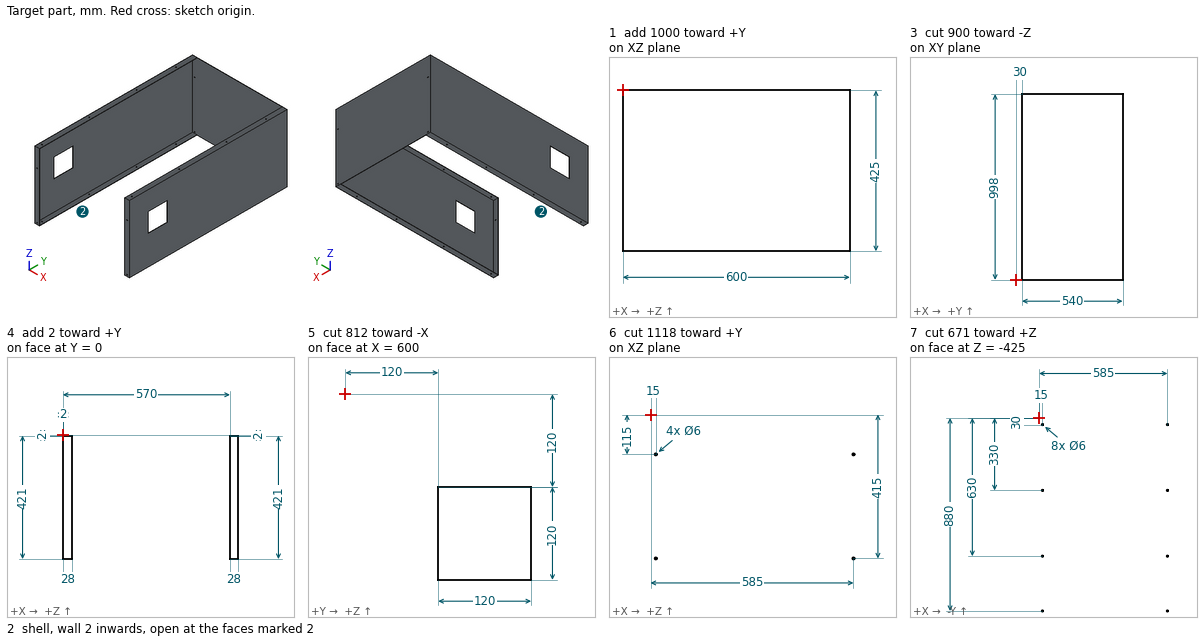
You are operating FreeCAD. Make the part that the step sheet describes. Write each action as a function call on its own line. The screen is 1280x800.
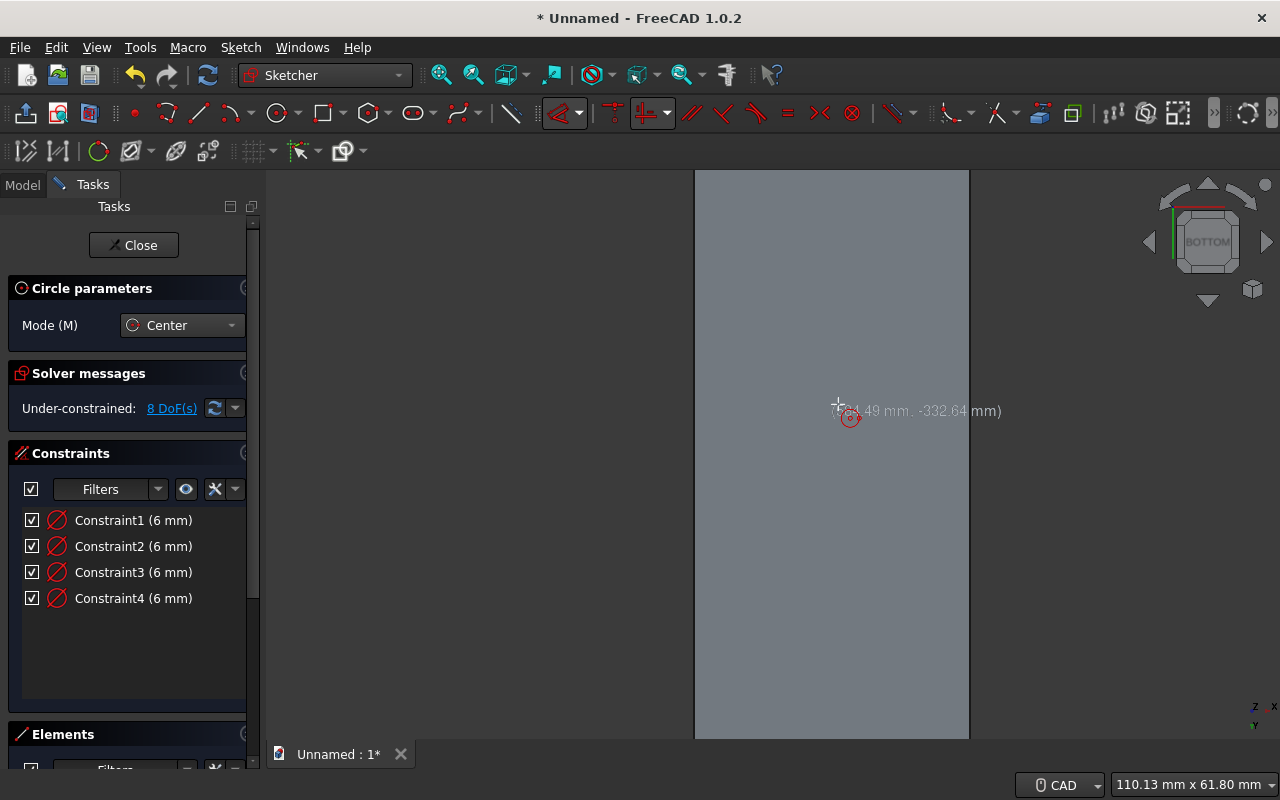
scroll(838, 404, down, 15)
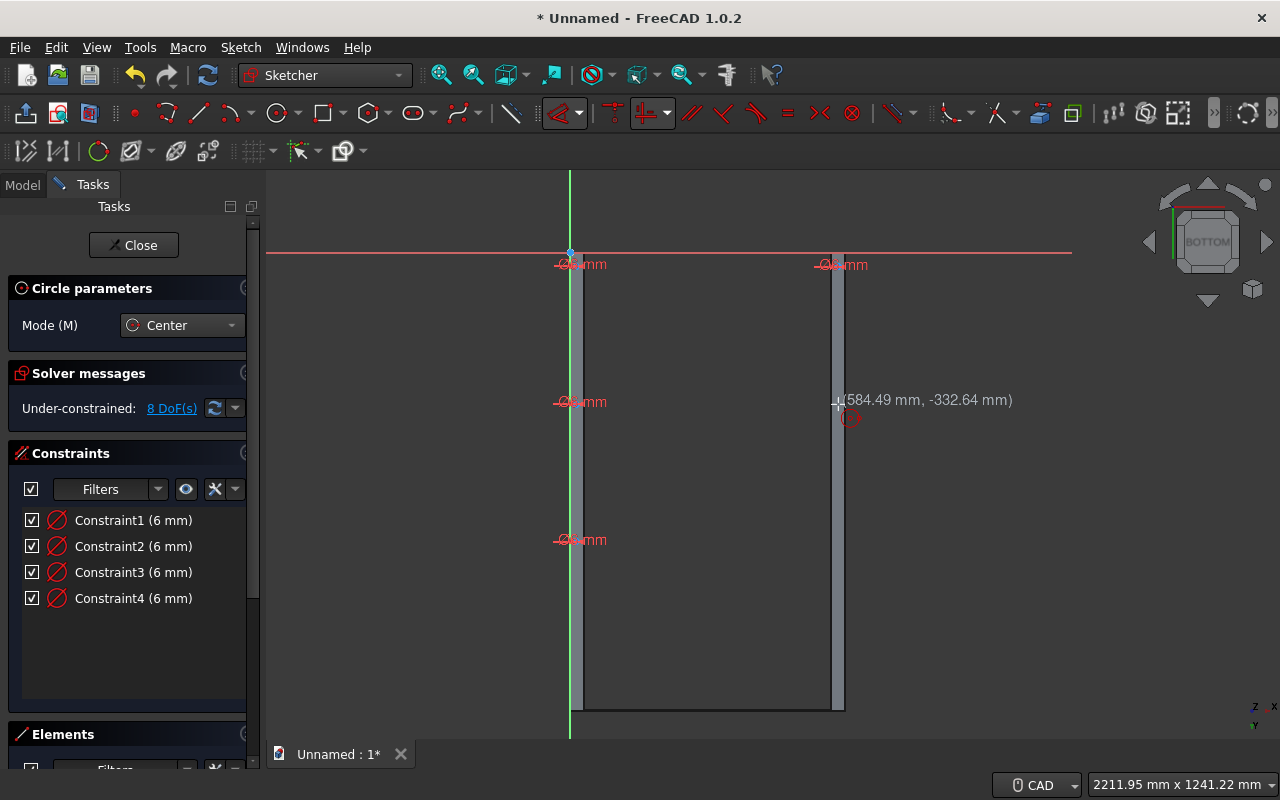
click(838, 404)
move(839, 403)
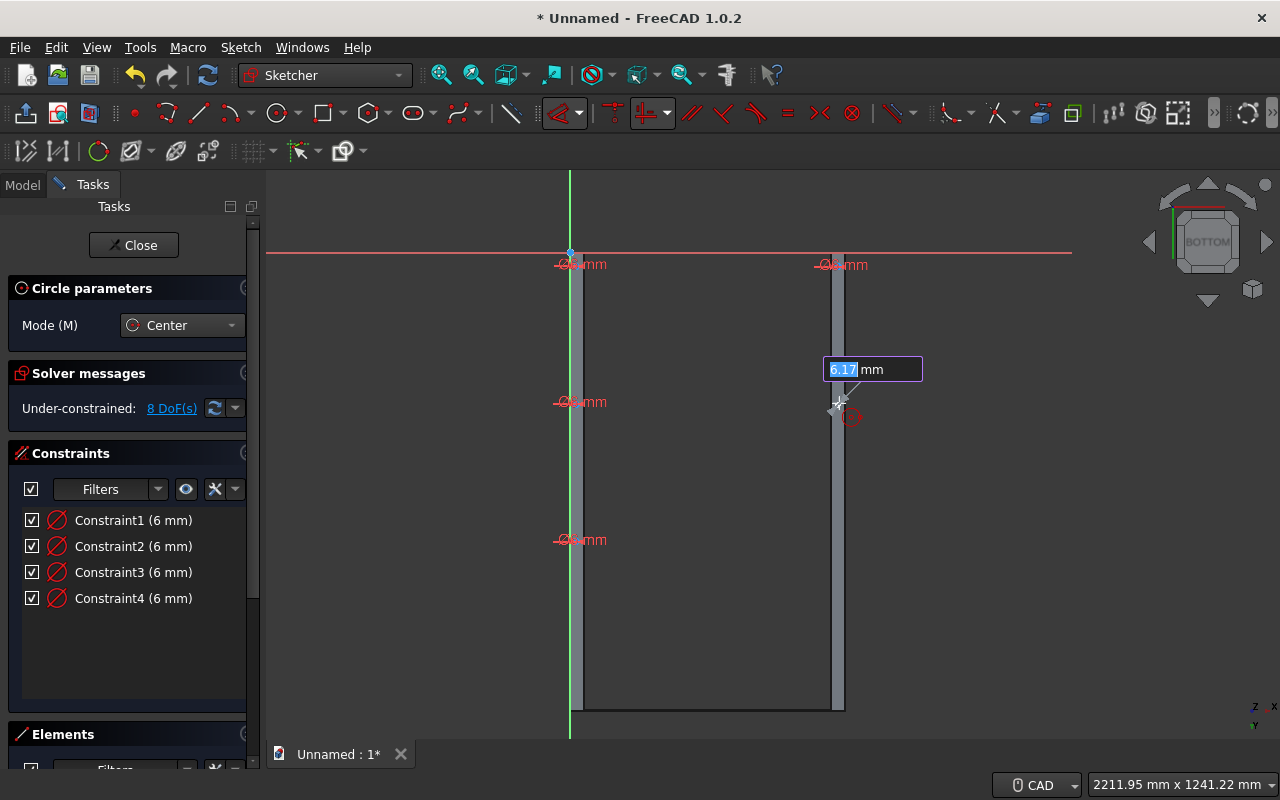
text(6)
key(Return)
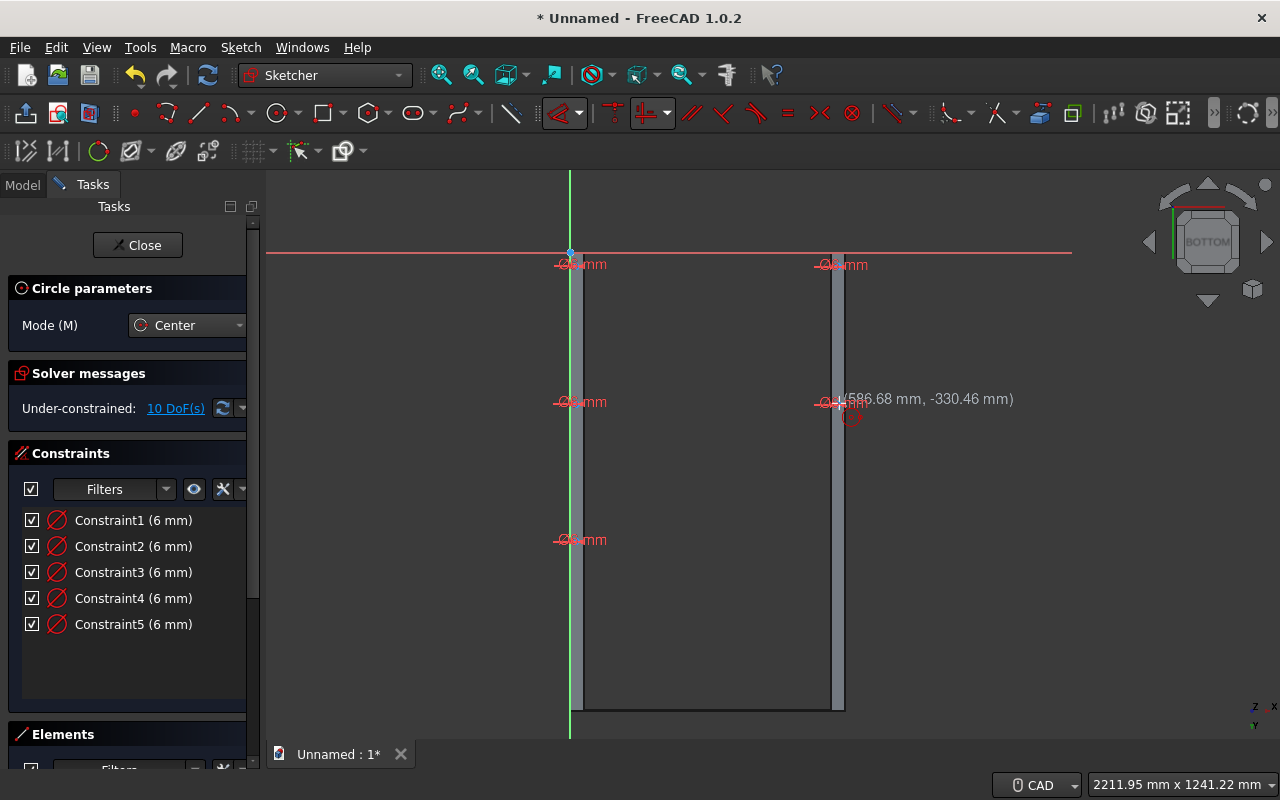
scroll(577, 656, up, 15)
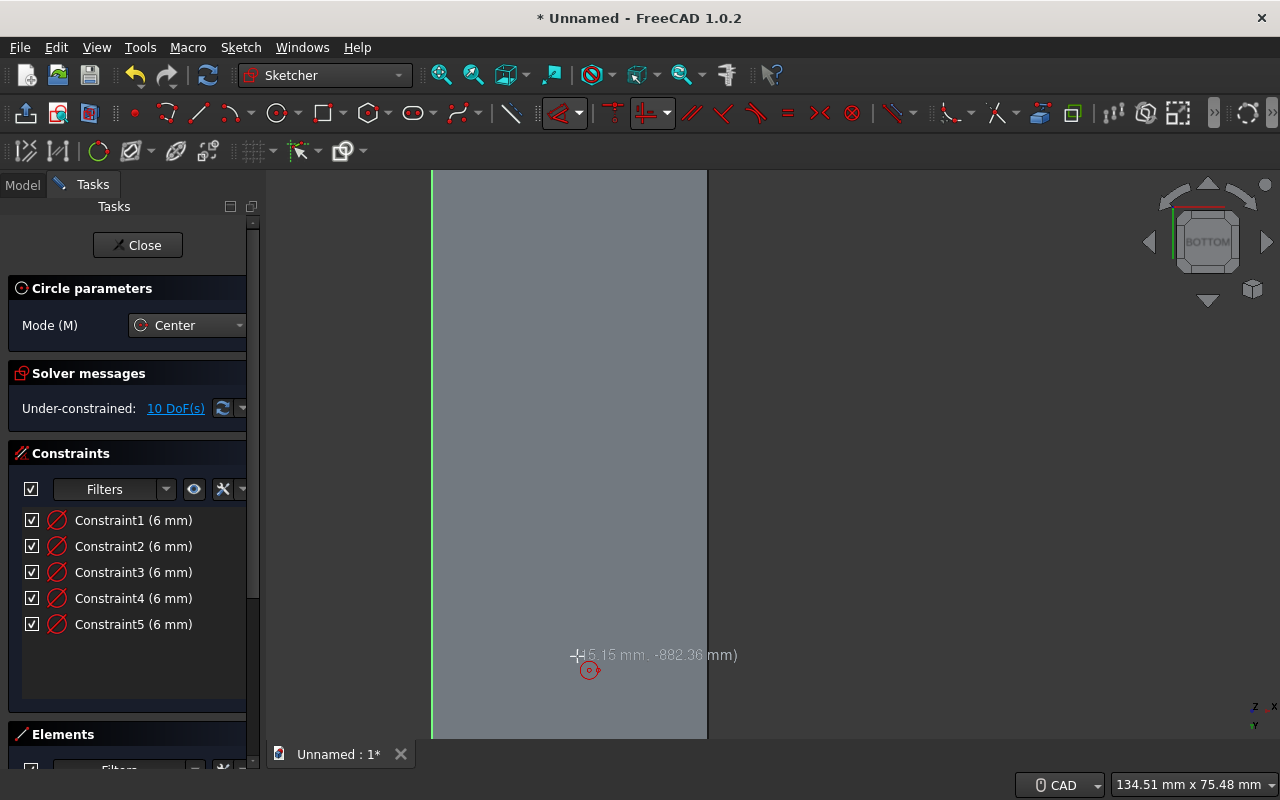
scroll(577, 656, down, 15)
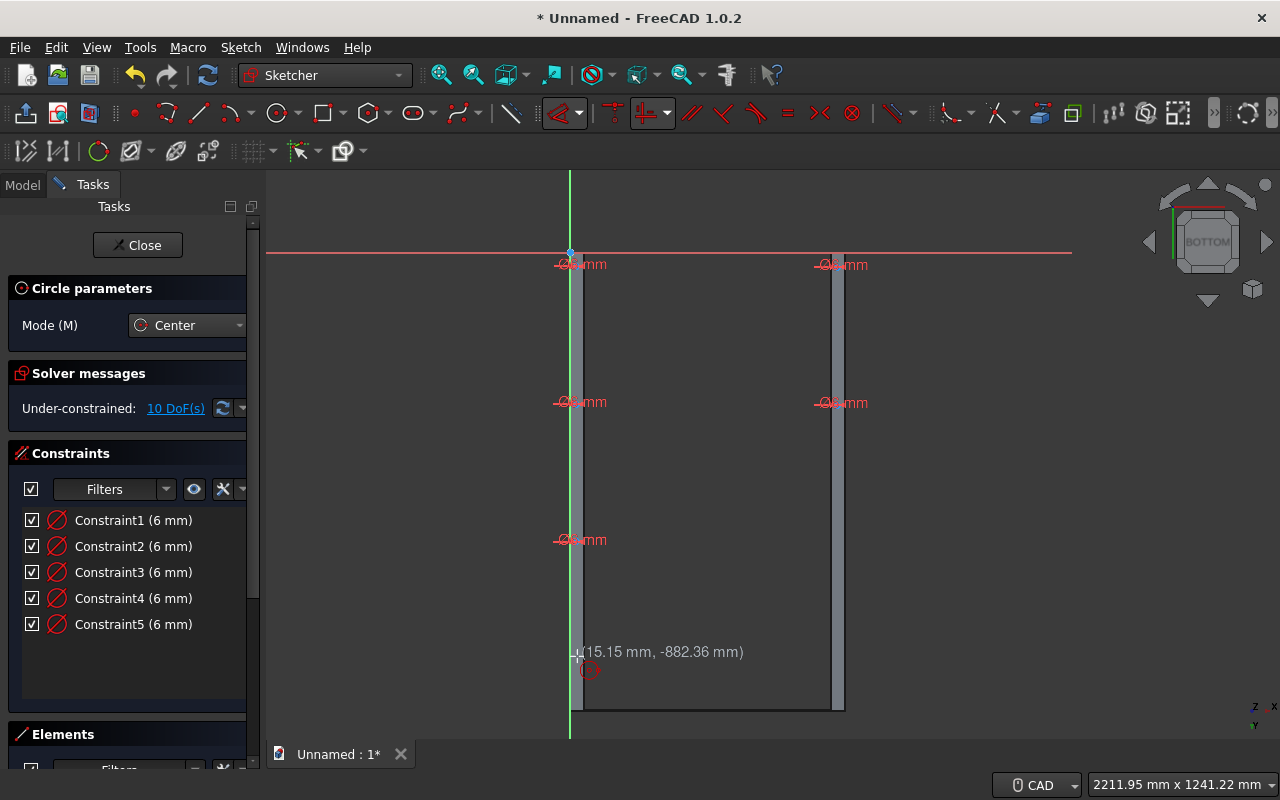
scroll(577, 656, up, 5)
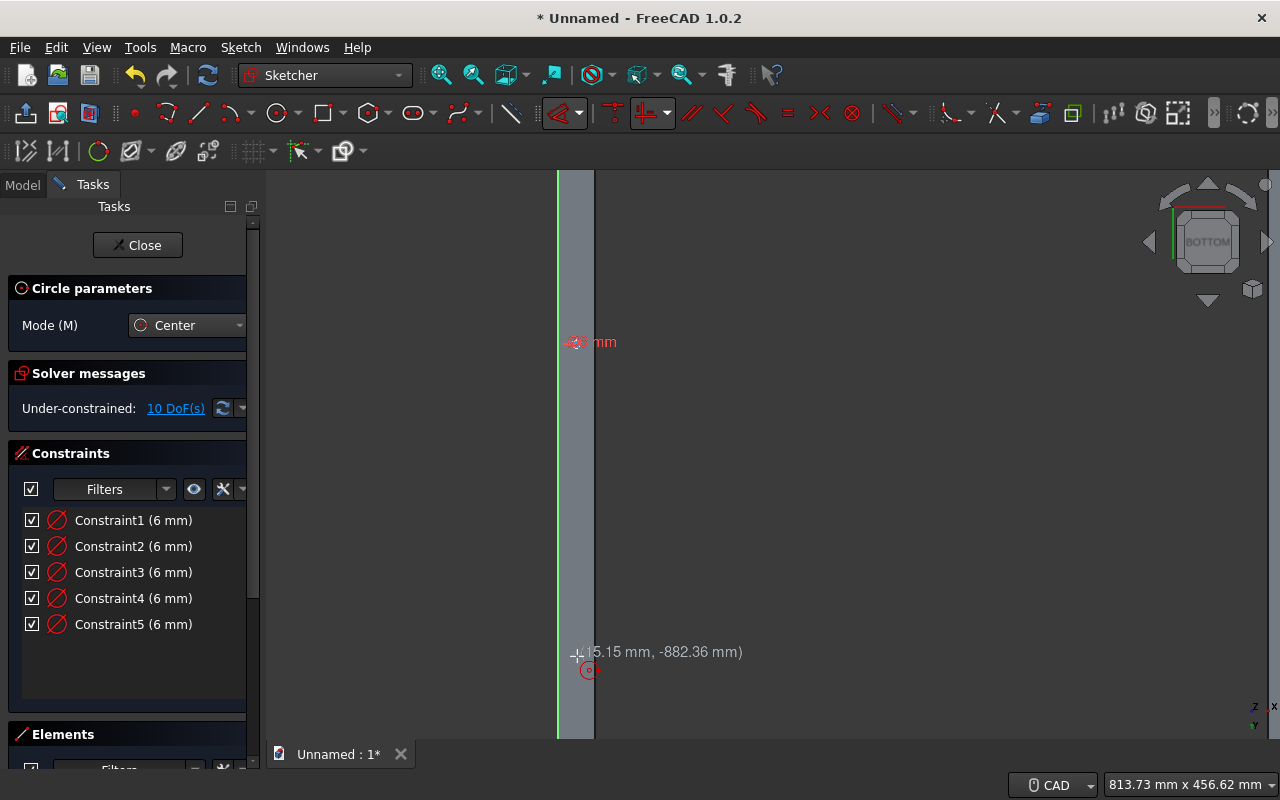
click(576, 654)
move(579, 652)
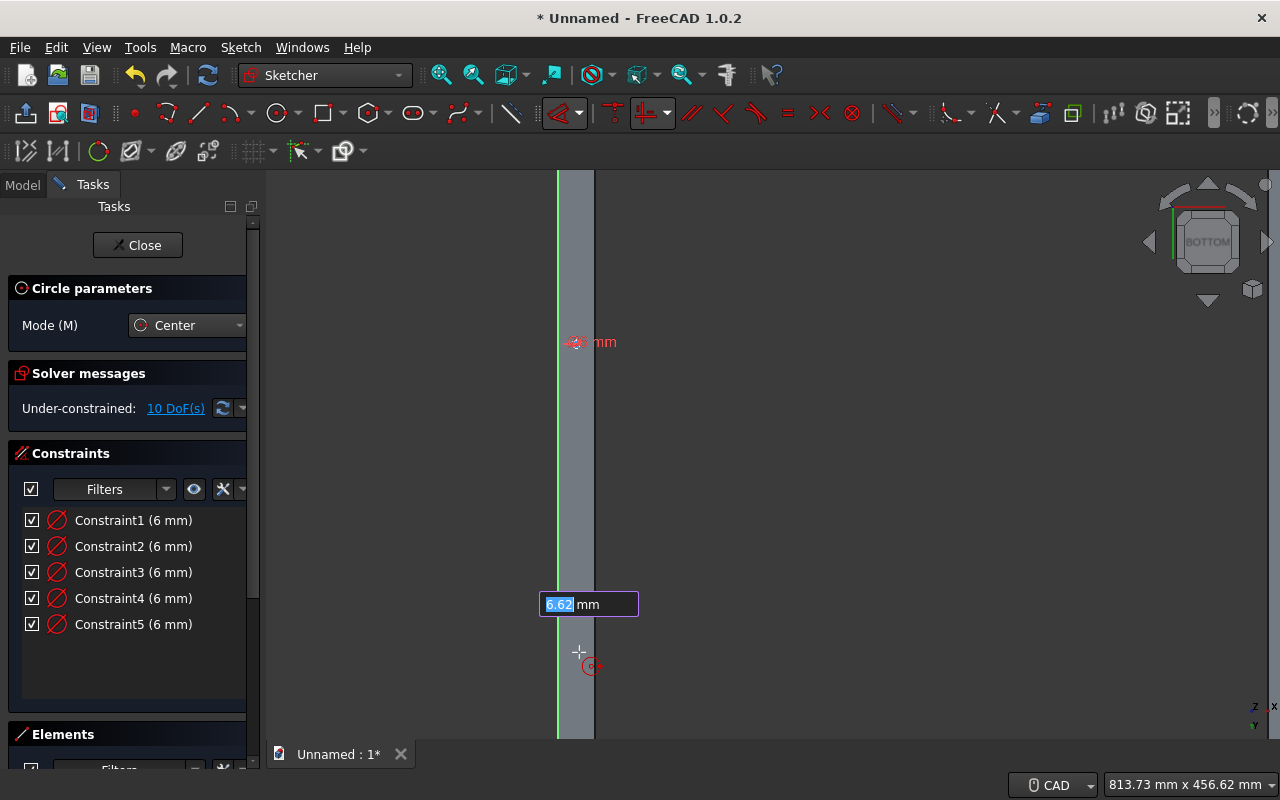
text(6)
key(Return)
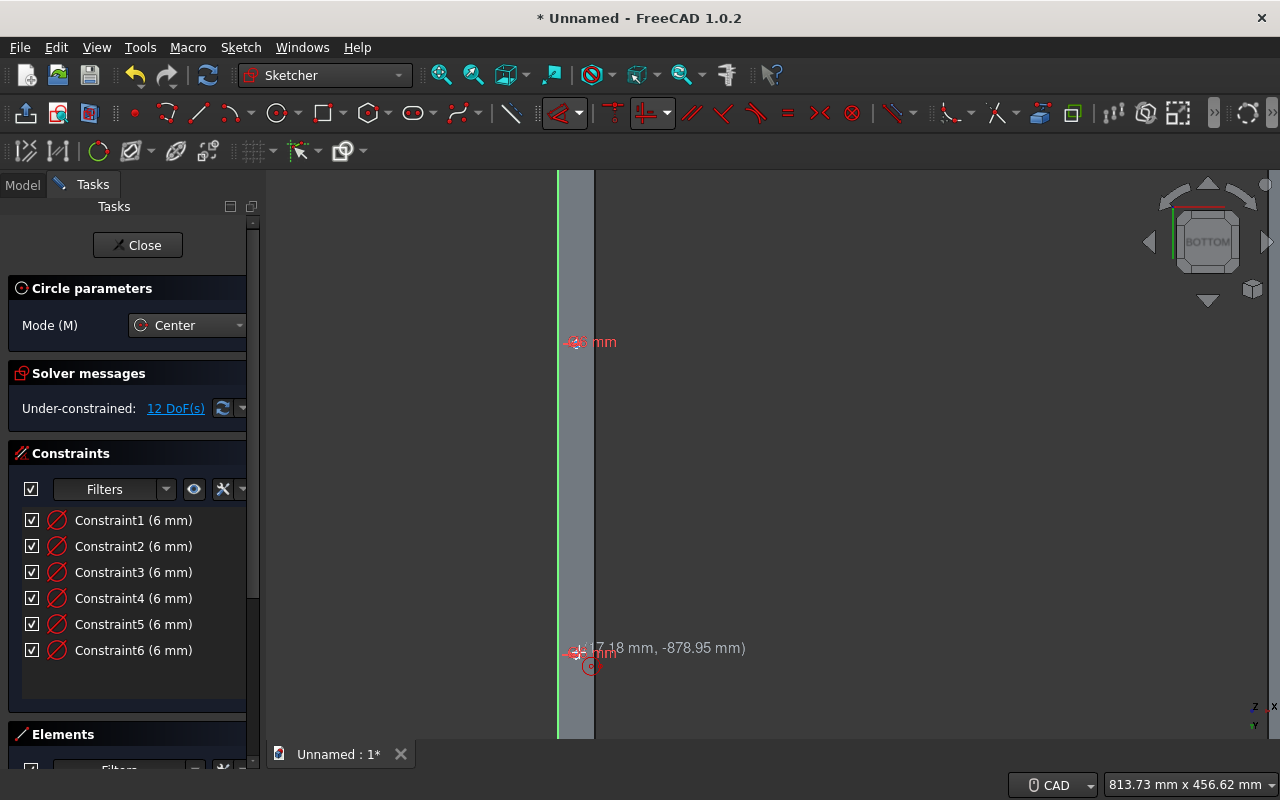
scroll(610, 604, down, 6)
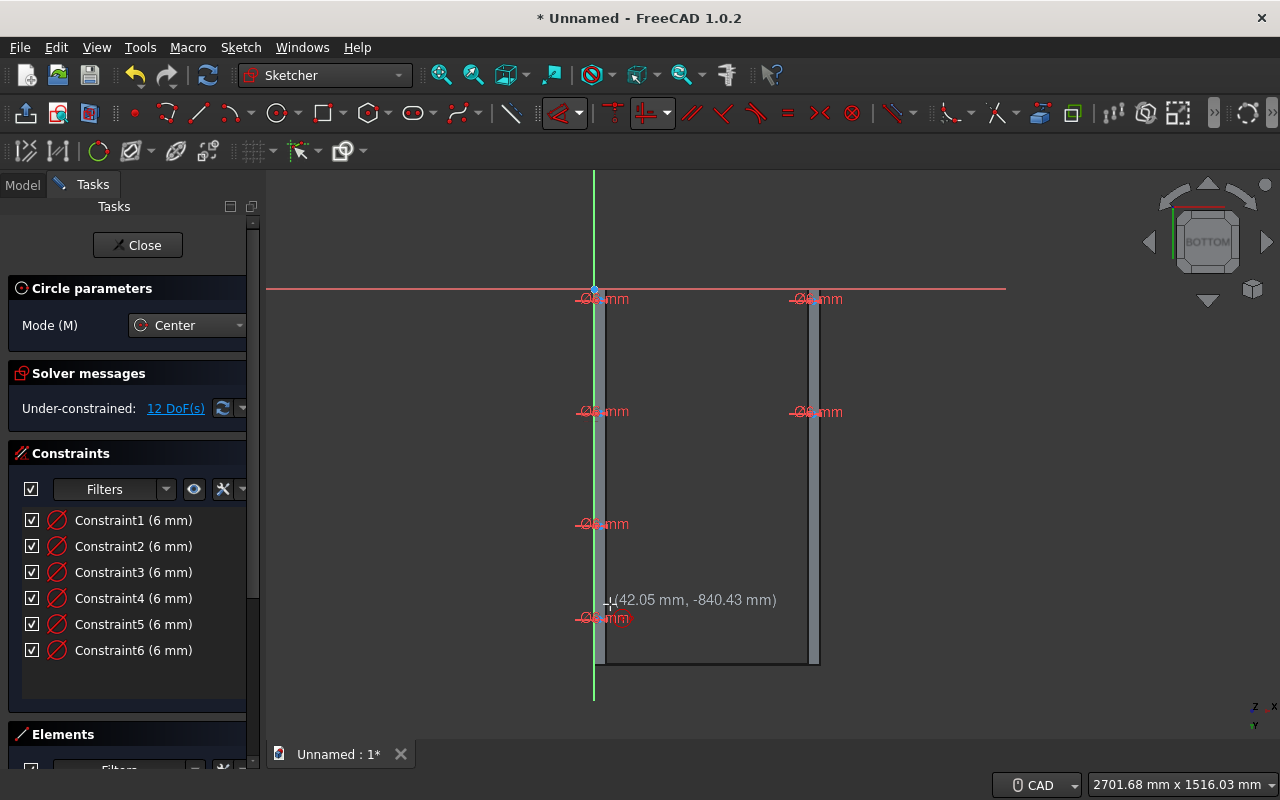
scroll(814, 526, up, 16)